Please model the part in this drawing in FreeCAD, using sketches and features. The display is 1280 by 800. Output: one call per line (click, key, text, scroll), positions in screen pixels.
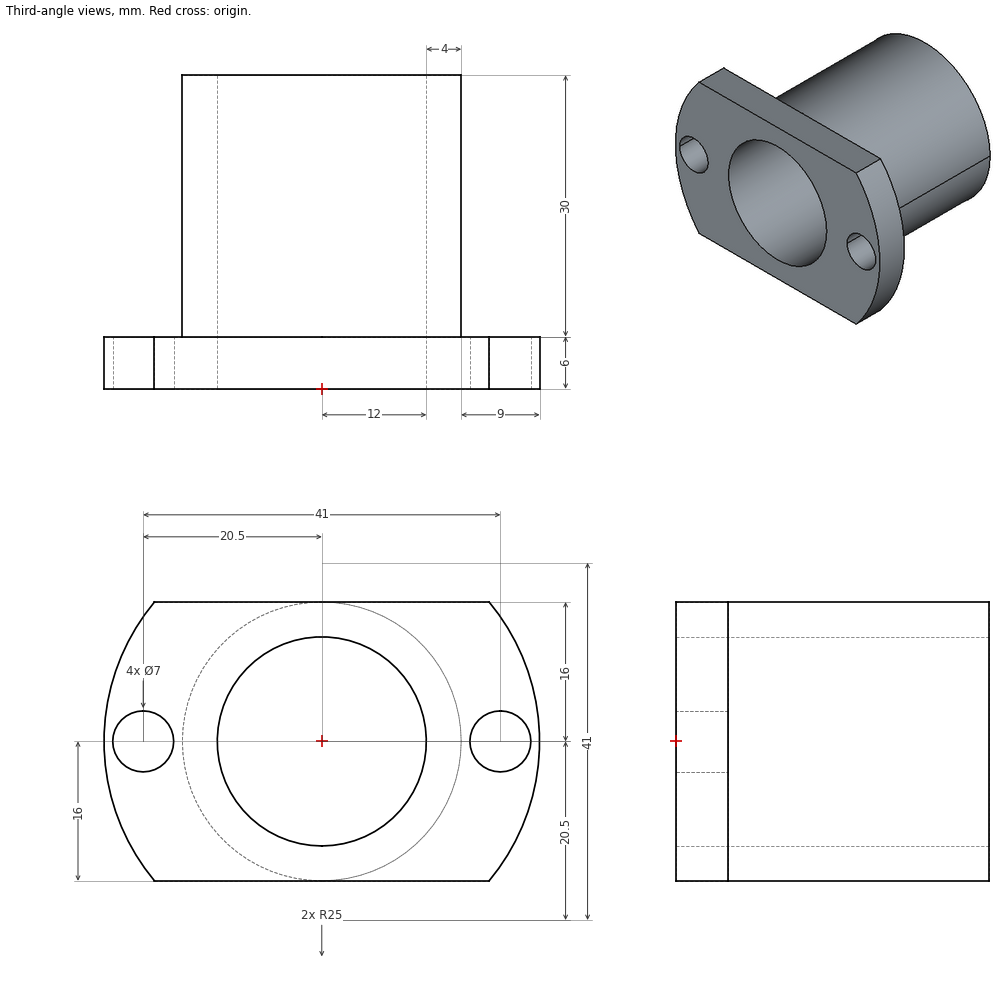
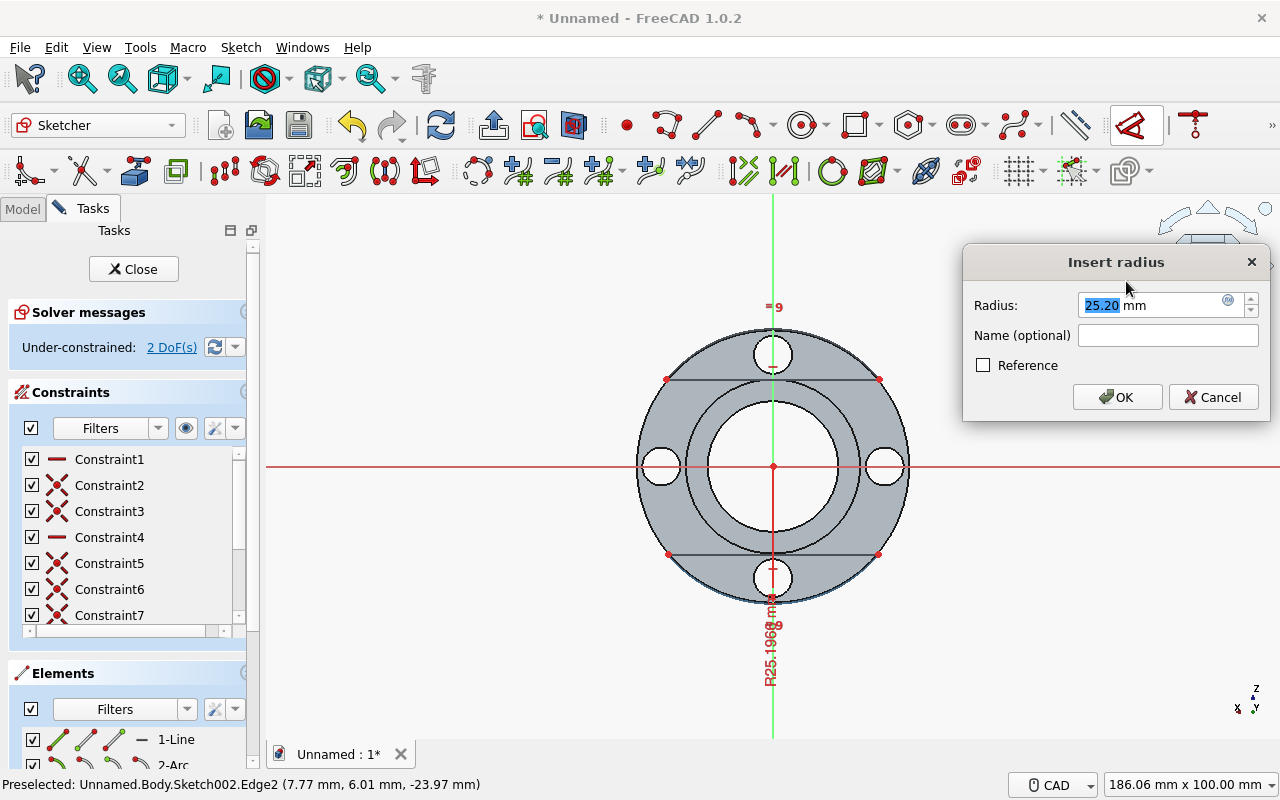
text(25)
key(Return)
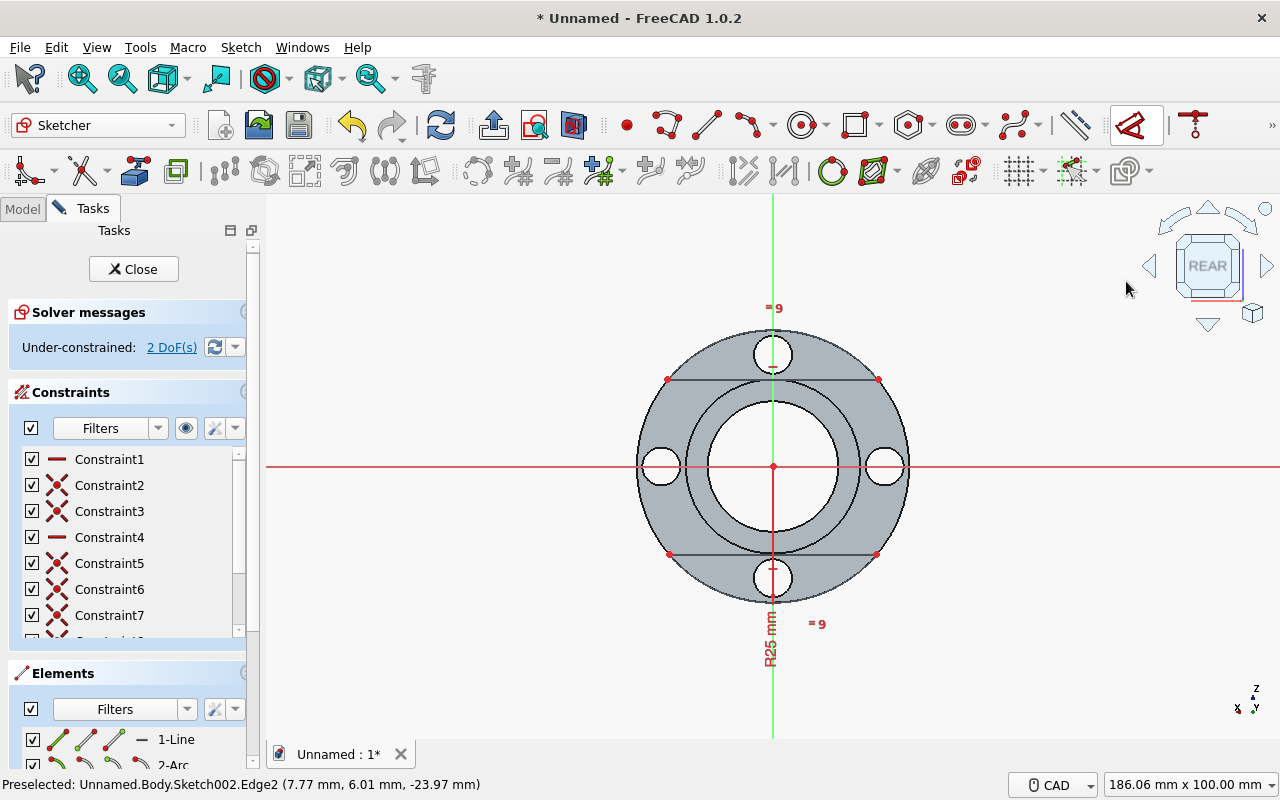
click(877, 555)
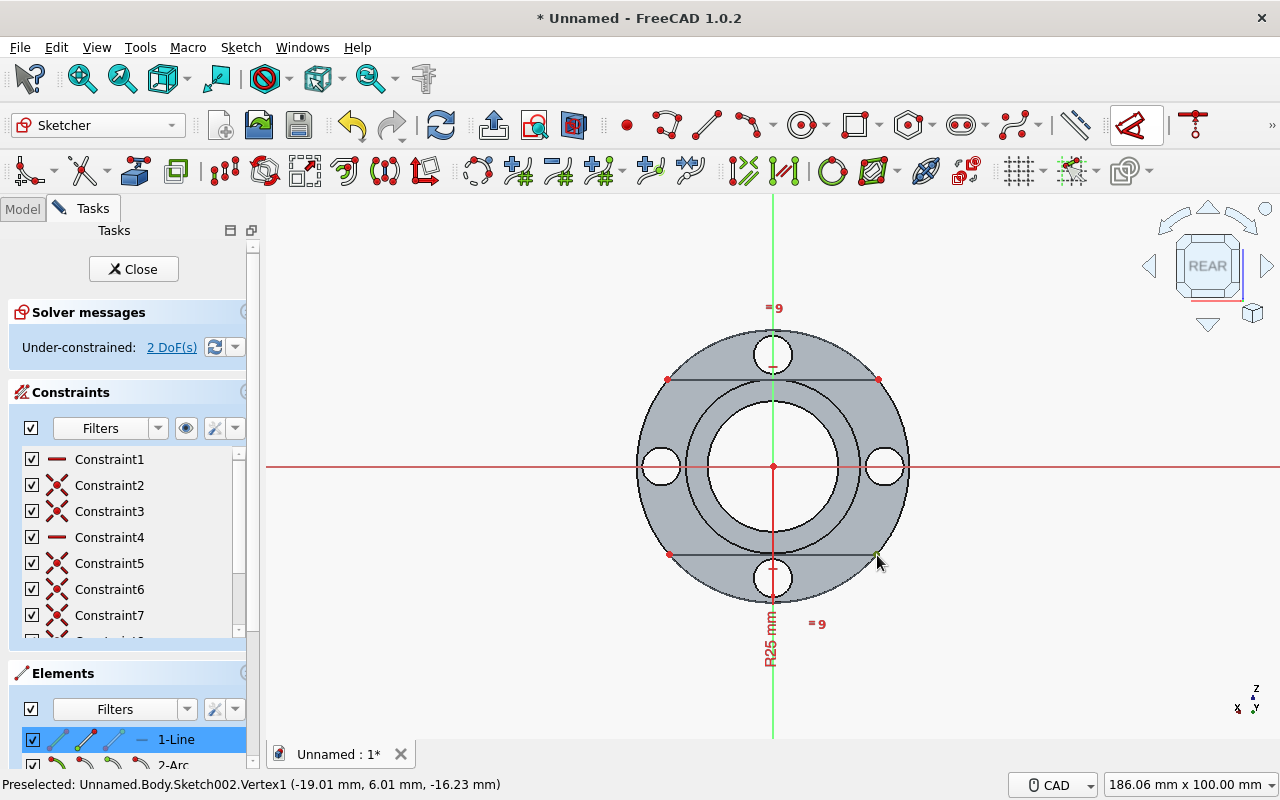
click(1158, 126)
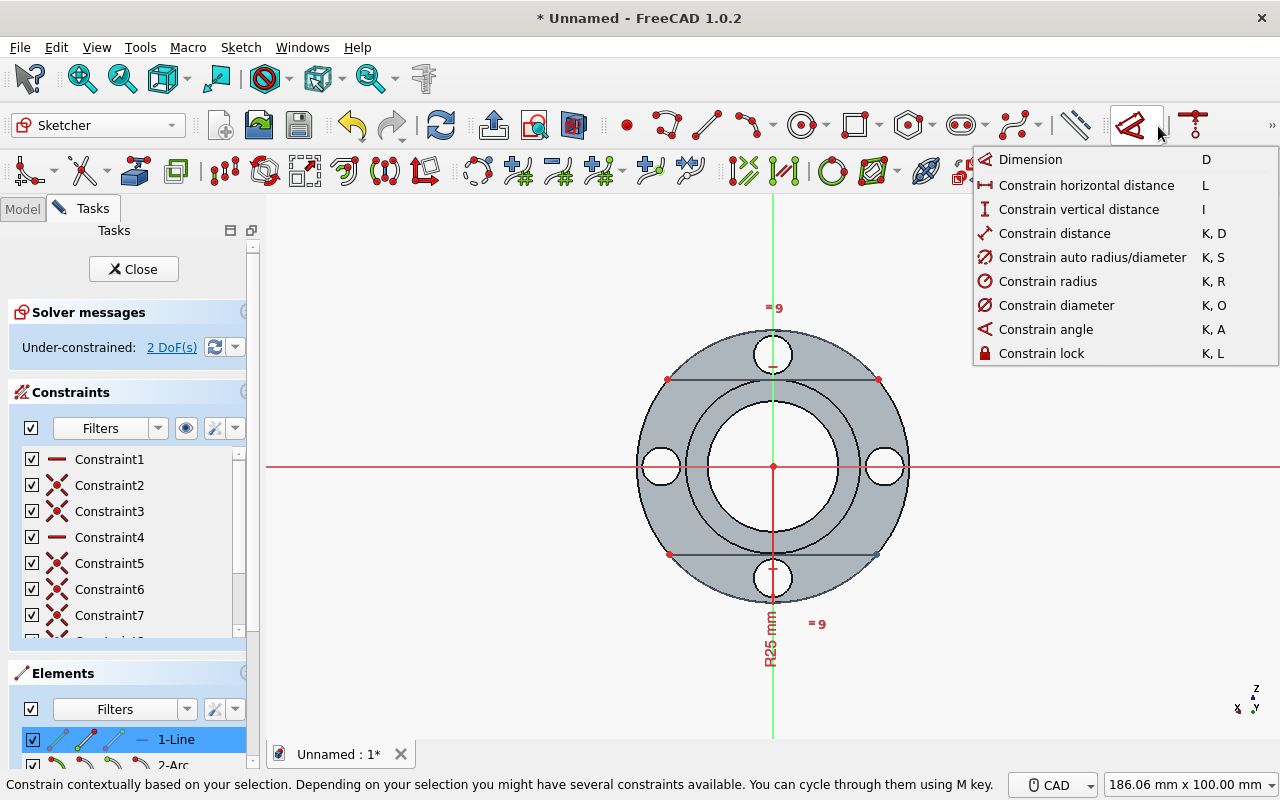
click(1126, 209)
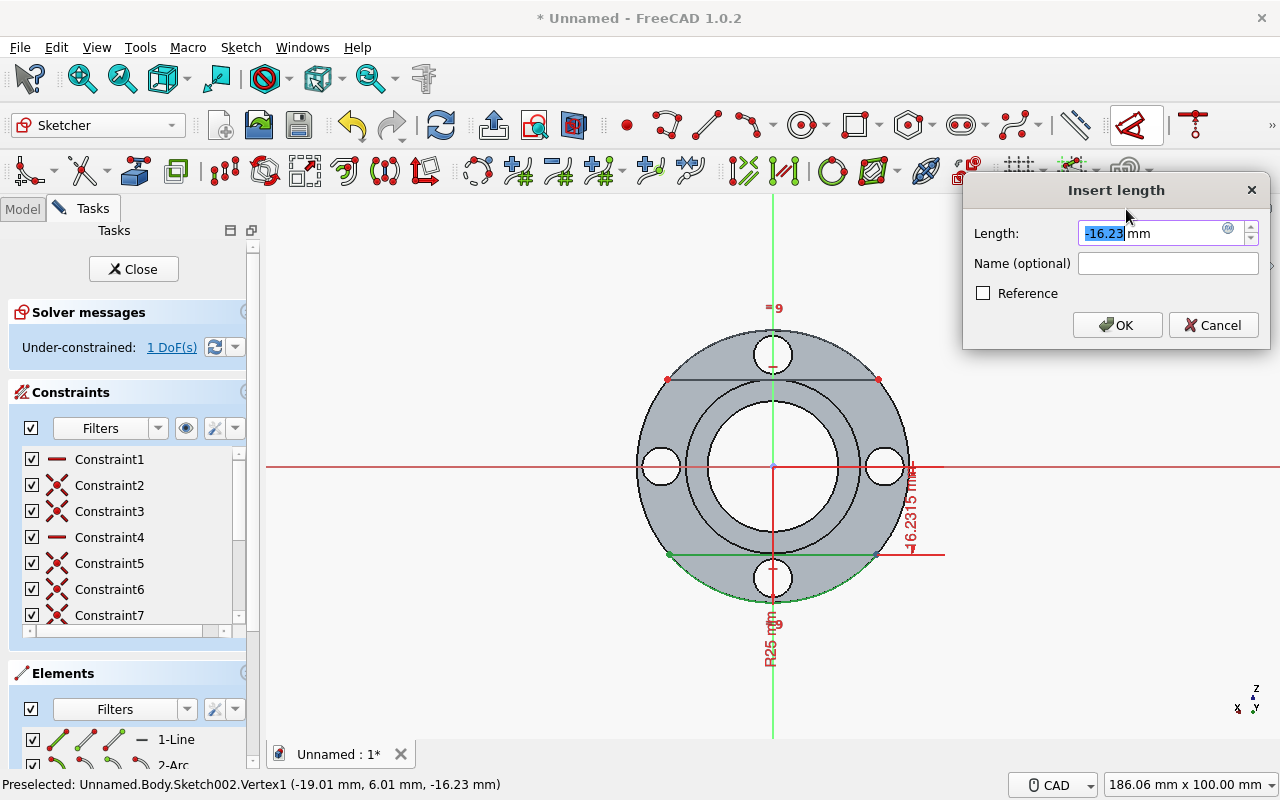
text(-16)
key(Return)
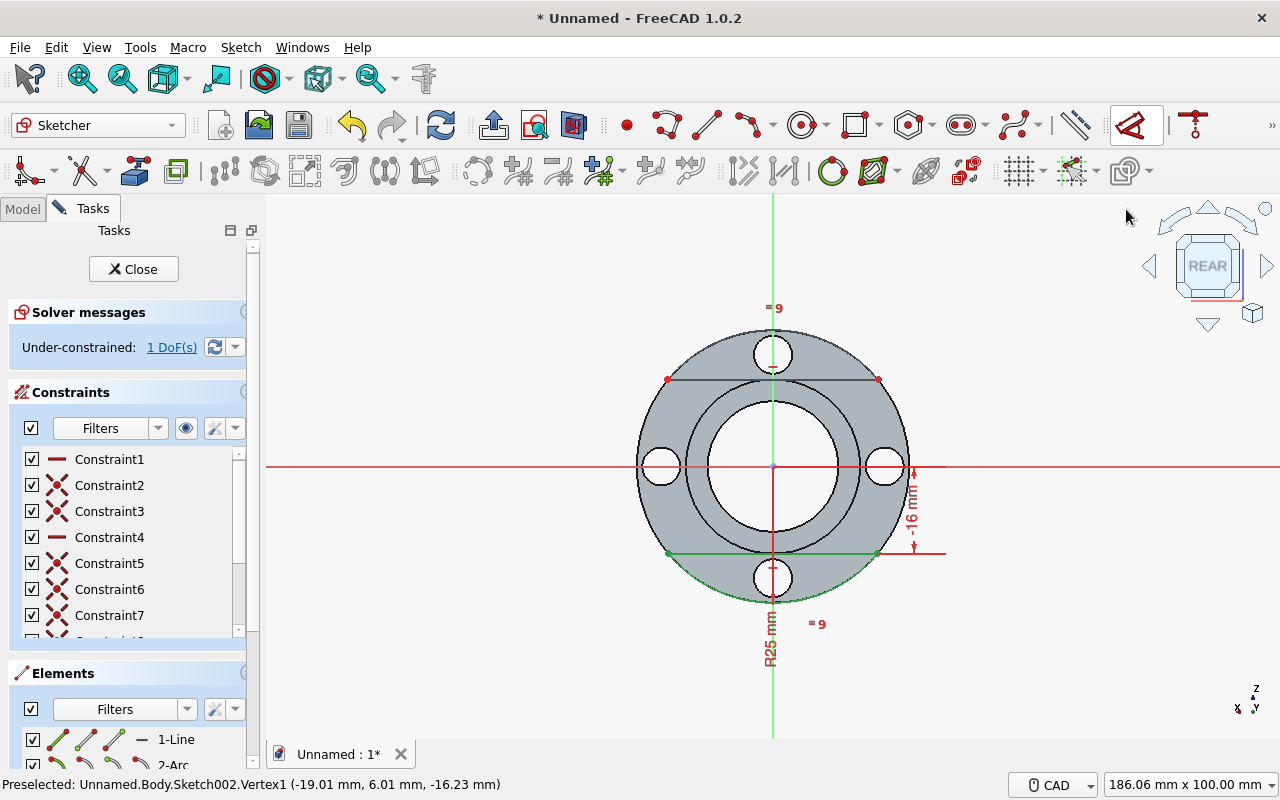
click(668, 380)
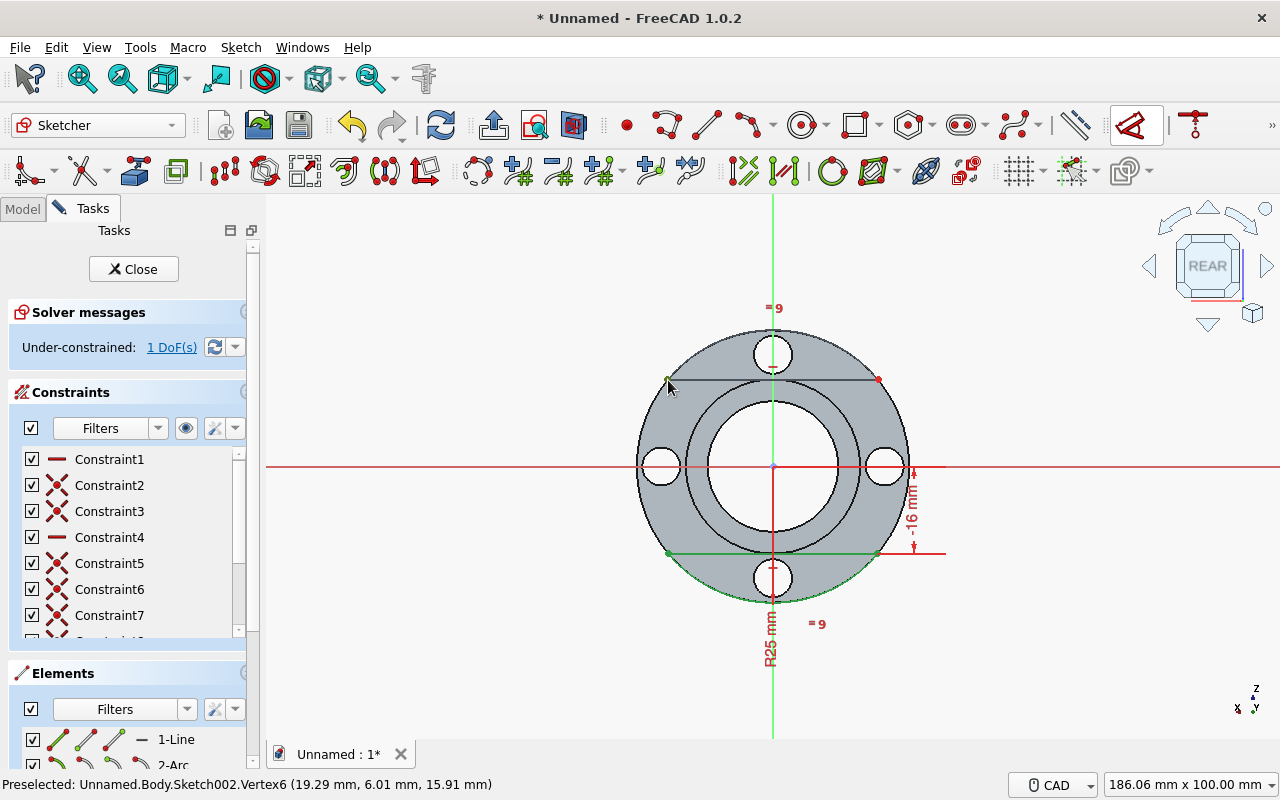
click(1158, 126)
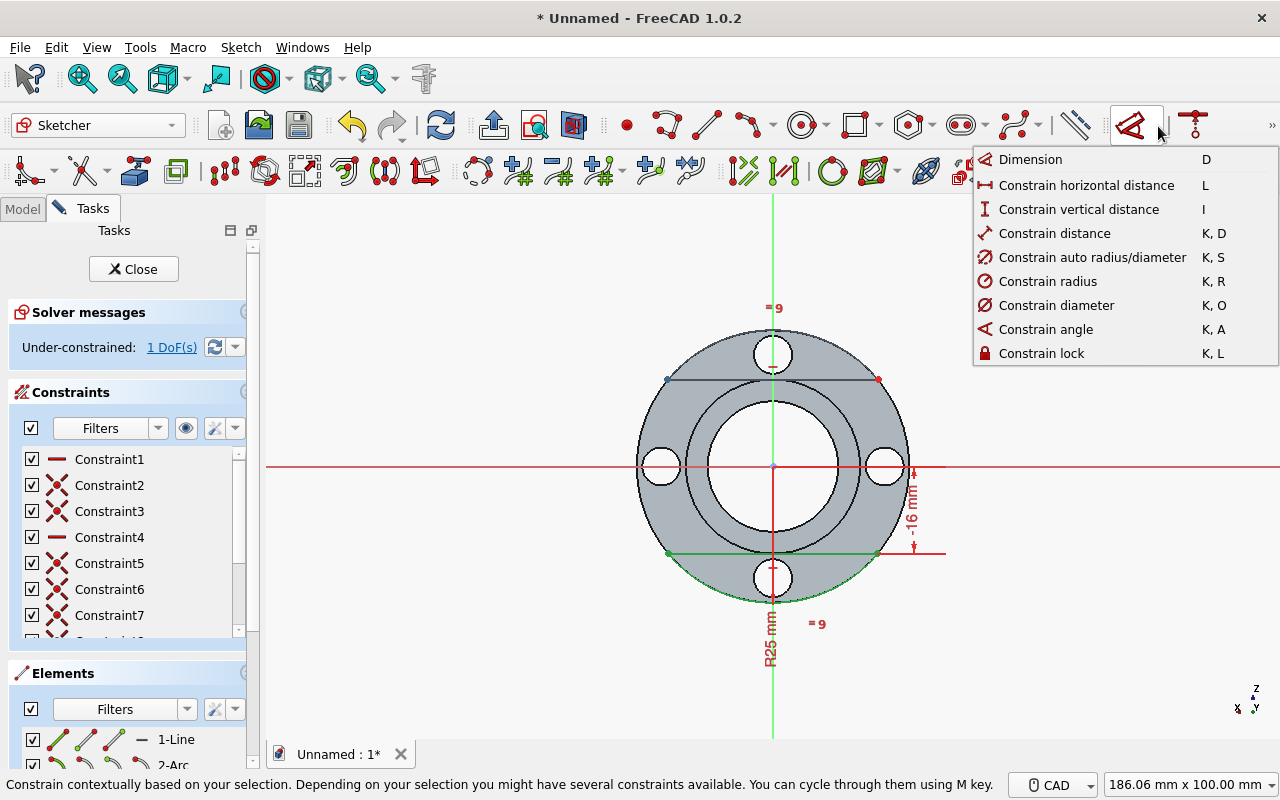
click(1126, 209)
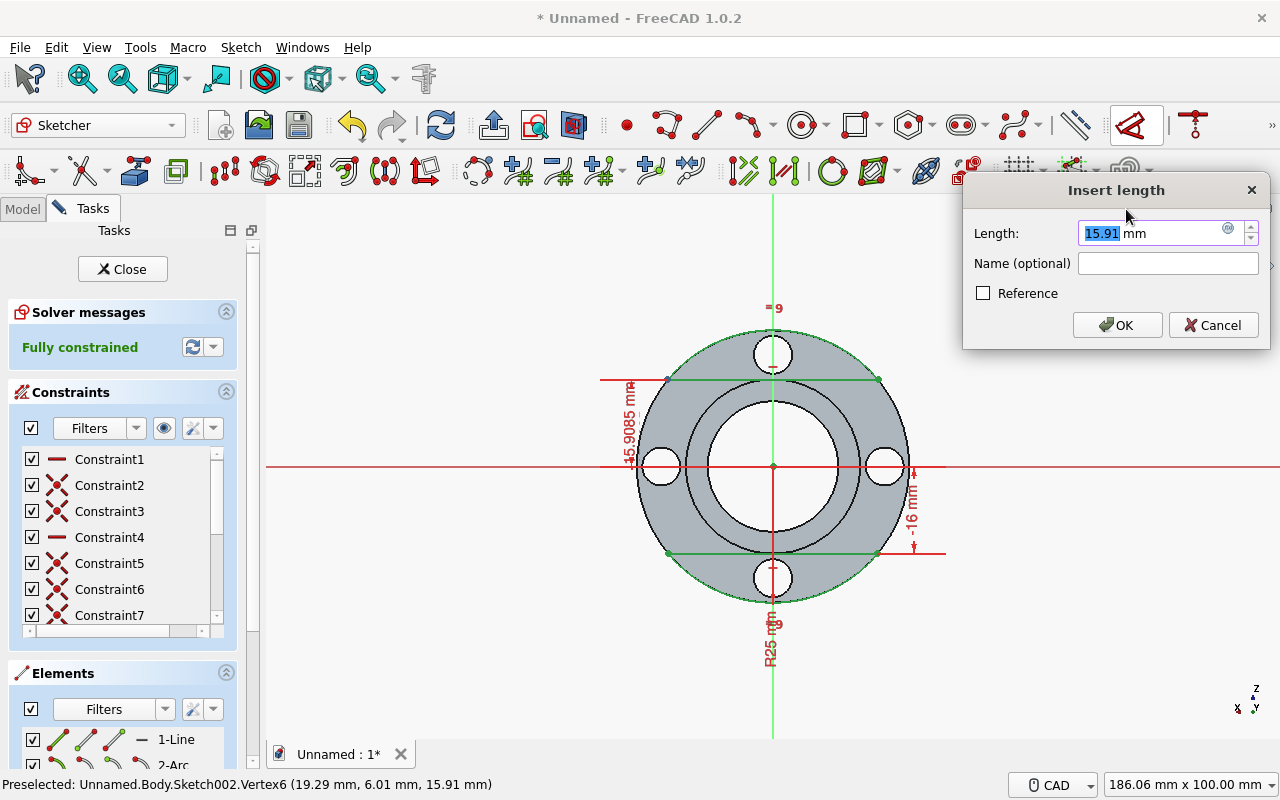
text(16)
key(Return)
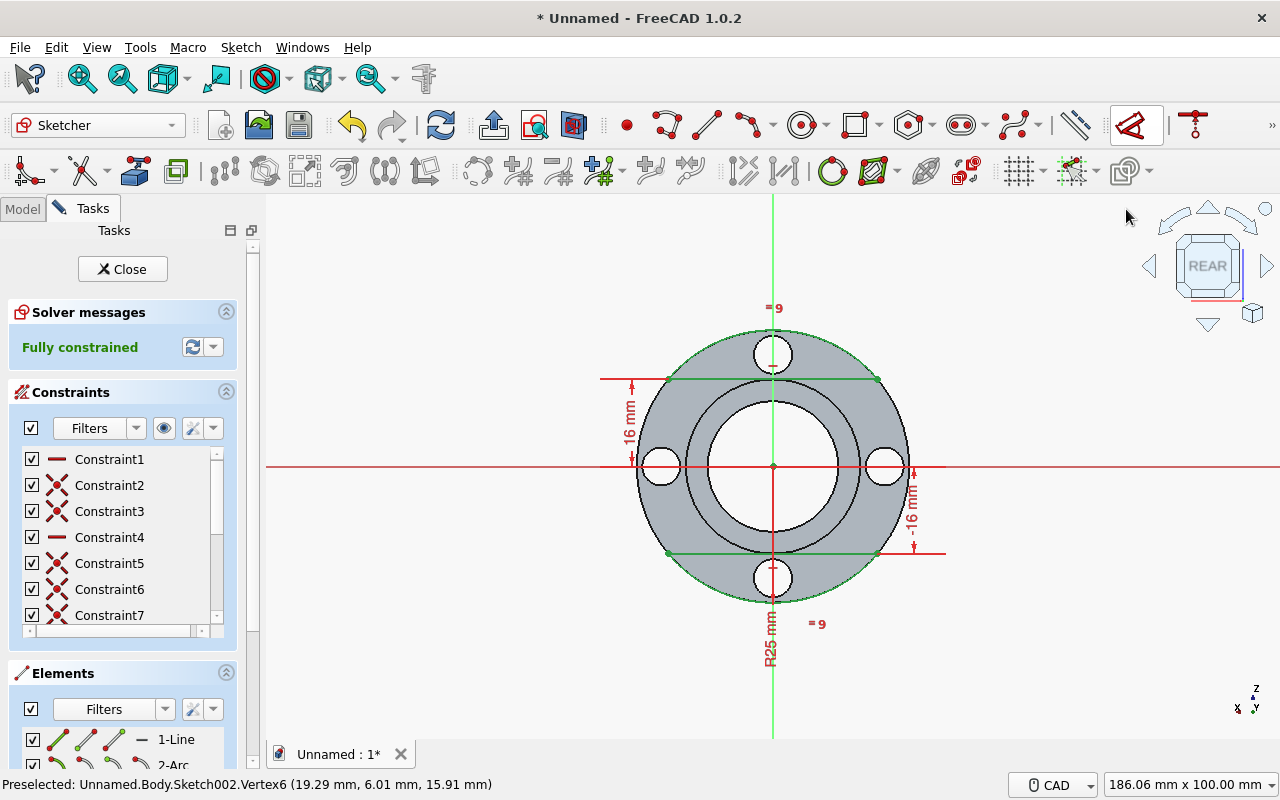
click(123, 269)